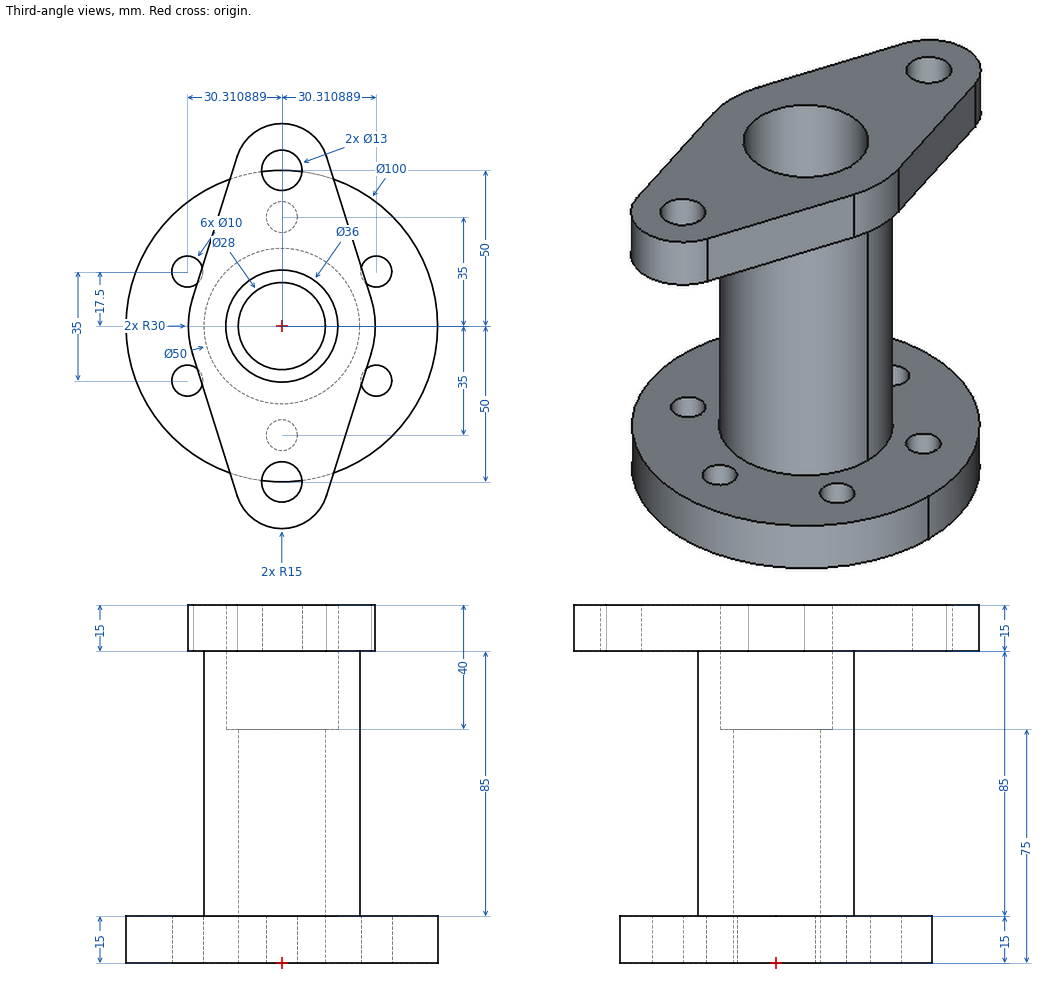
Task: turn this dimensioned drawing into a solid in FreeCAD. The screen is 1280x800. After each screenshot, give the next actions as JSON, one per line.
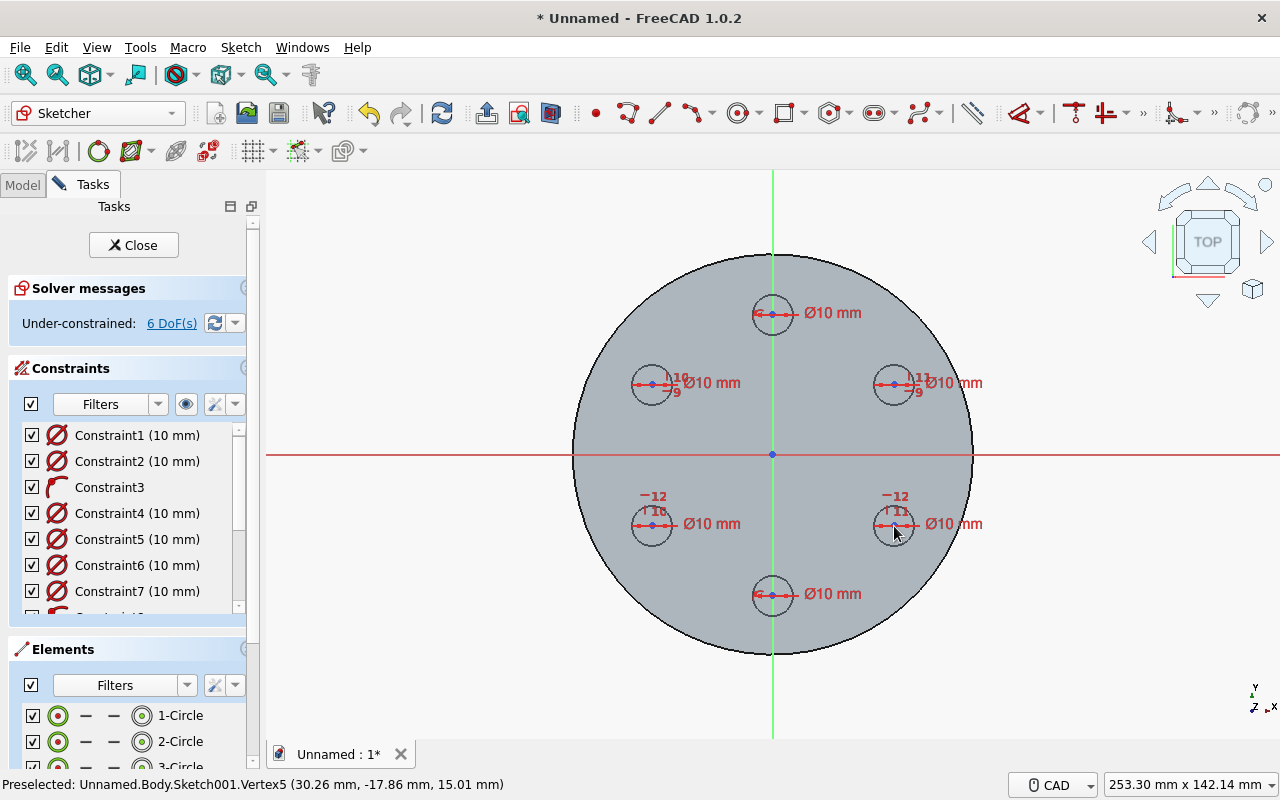
{"action": "left_click", "coordinate": [773, 315]}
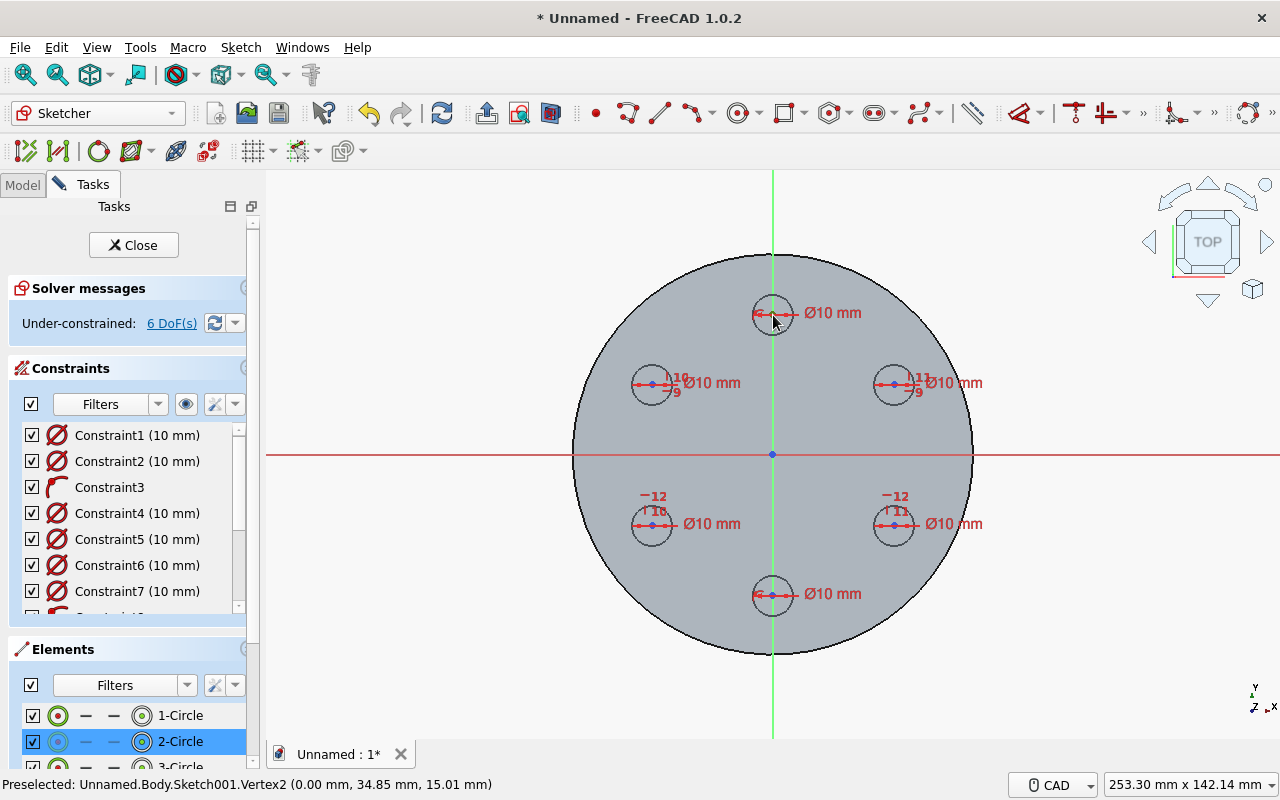
{"action": "key", "text": "i"}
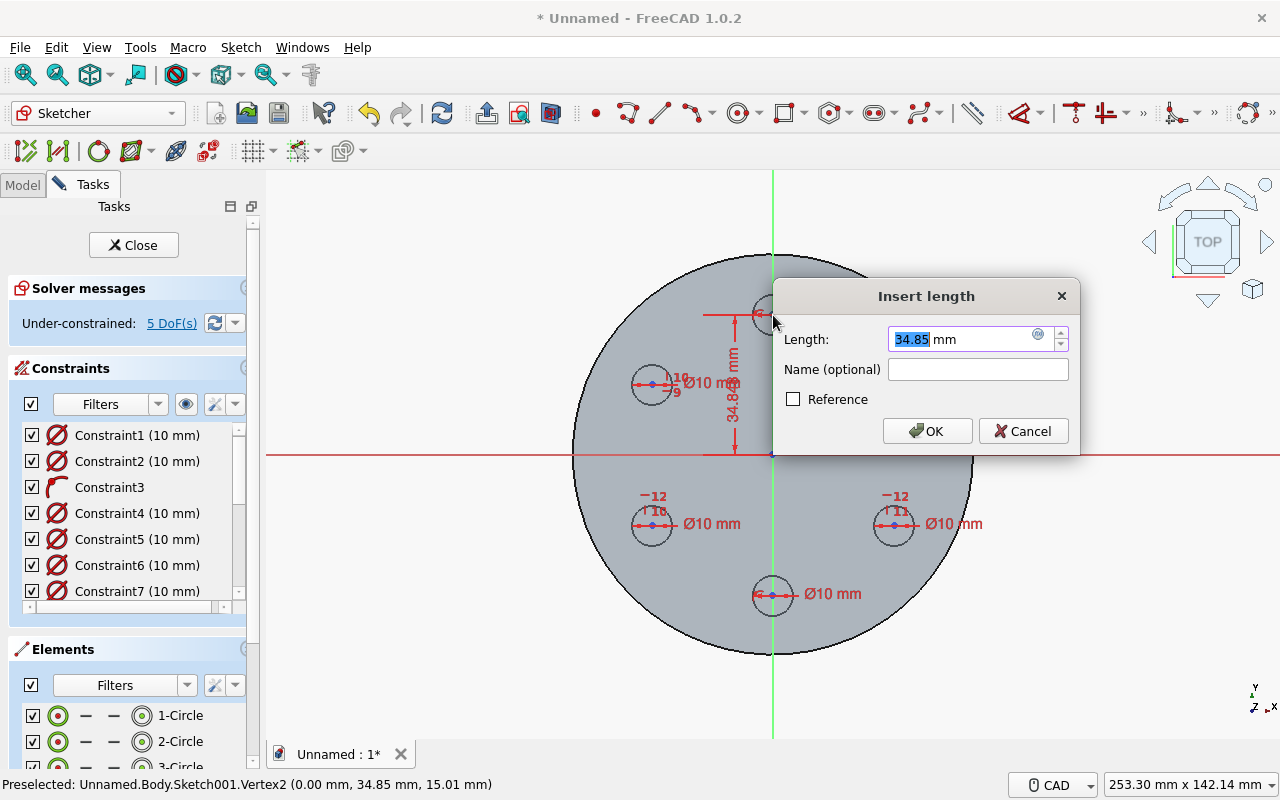
{"action": "type", "text": "35"}
{"action": "key", "text": "Return"}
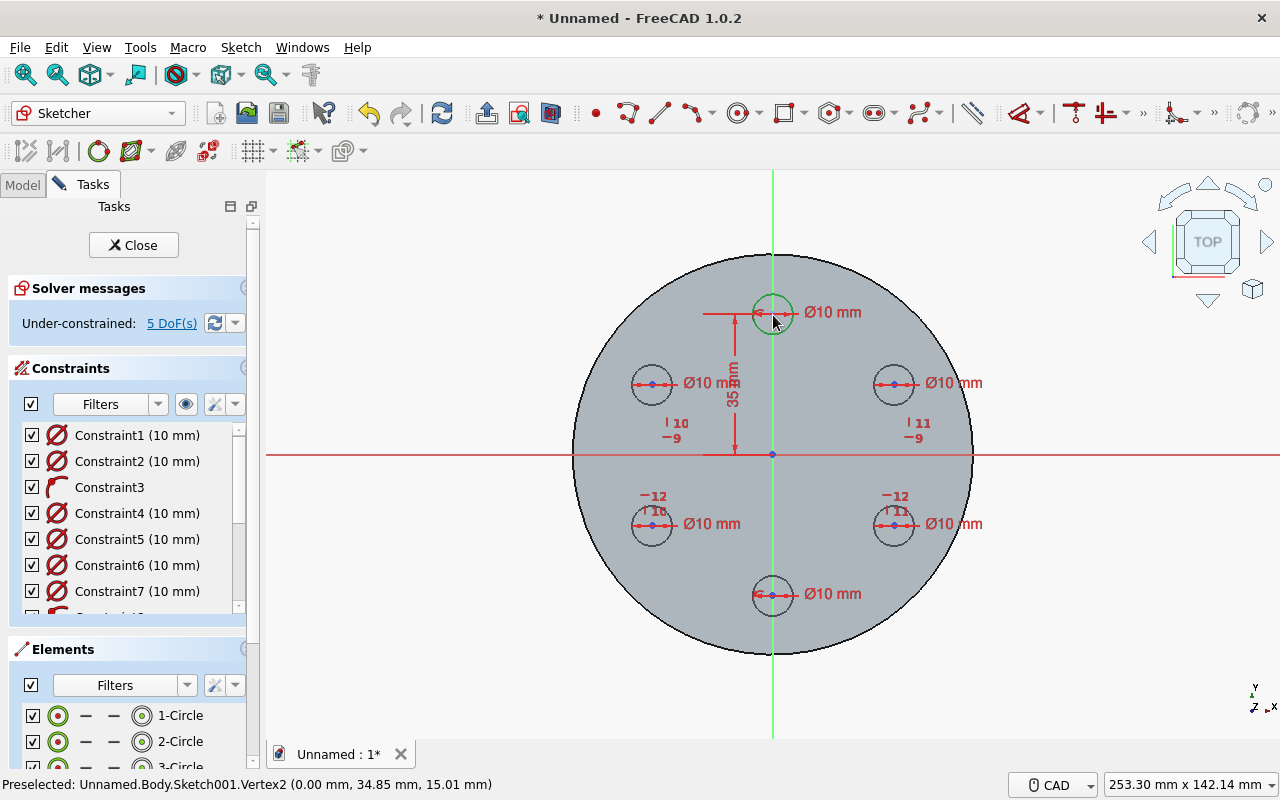
{"action": "left_click", "coordinate": [773, 596]}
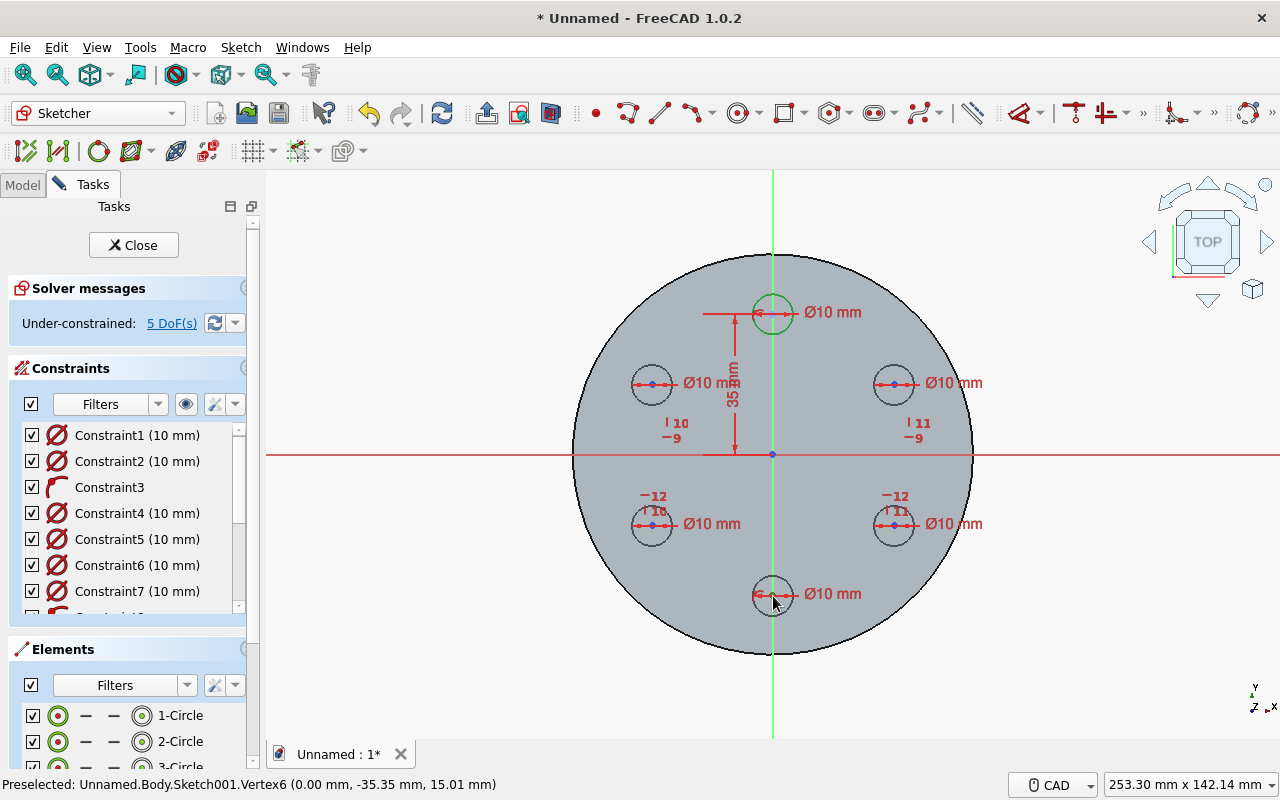
{"action": "key", "text": "i"}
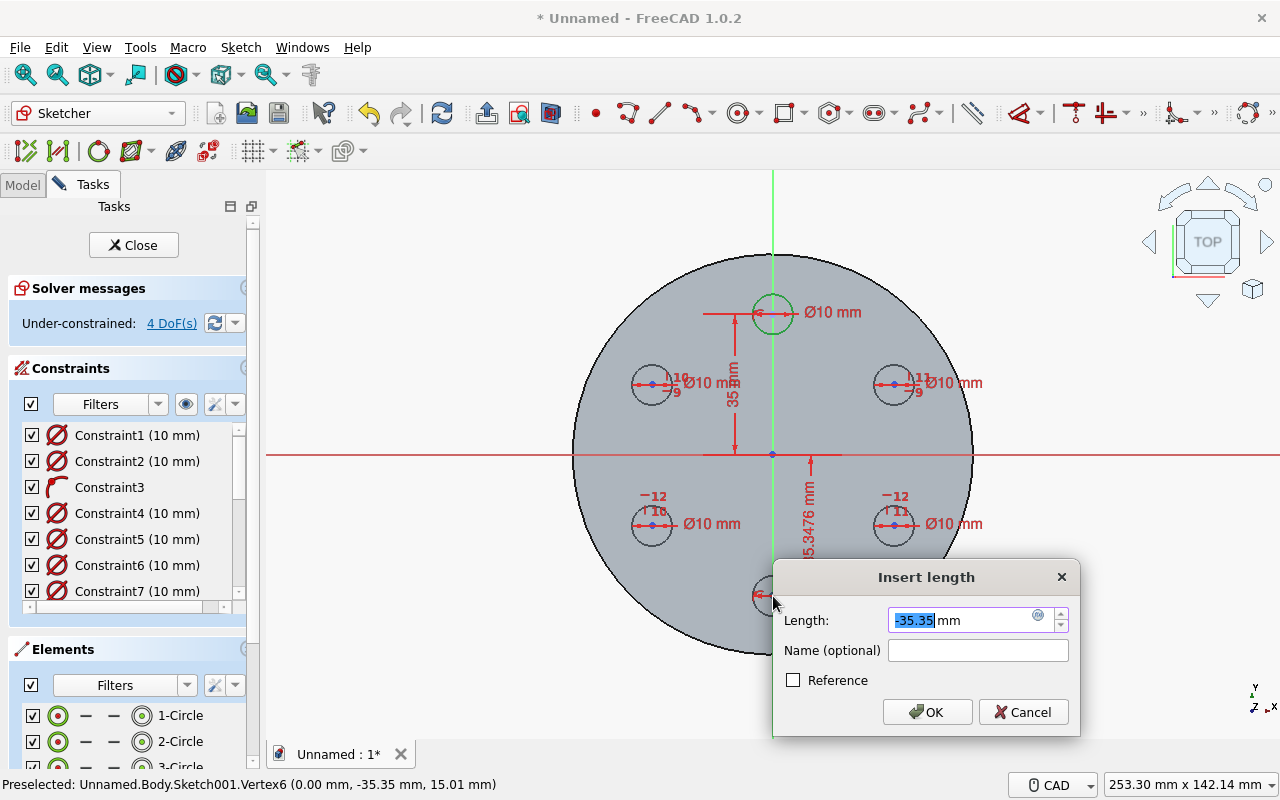
{"action": "type", "text": "-35"}
{"action": "key", "text": "Return"}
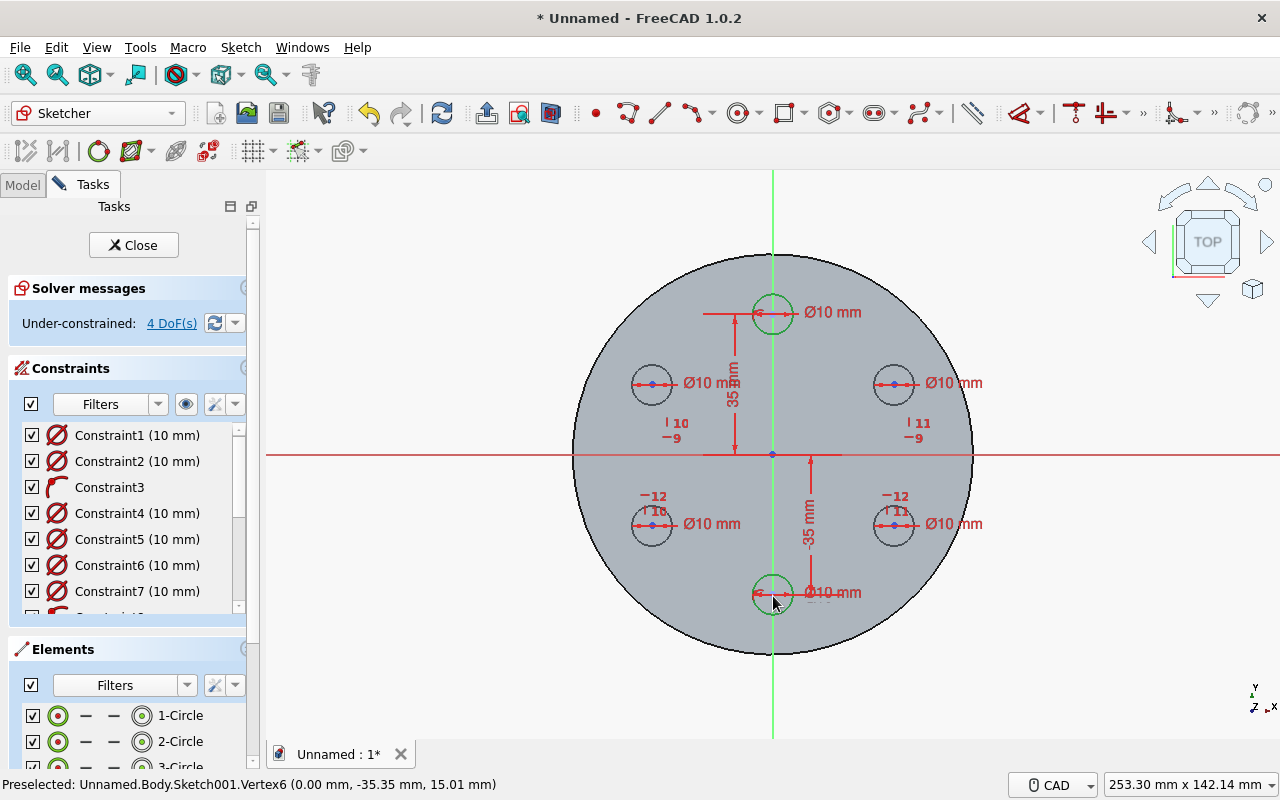
{"action": "left_click", "coordinate": [652, 385]}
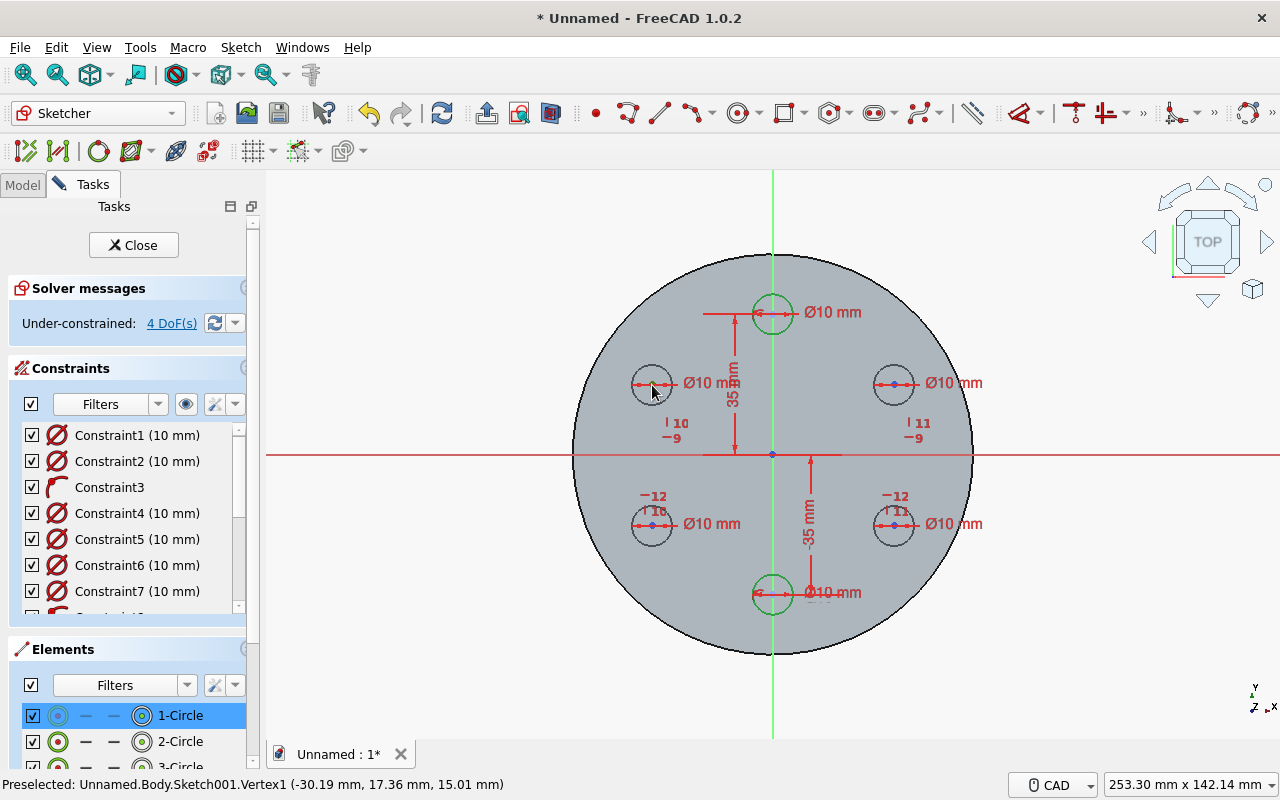
{"action": "left_click", "coordinate": [652, 526]}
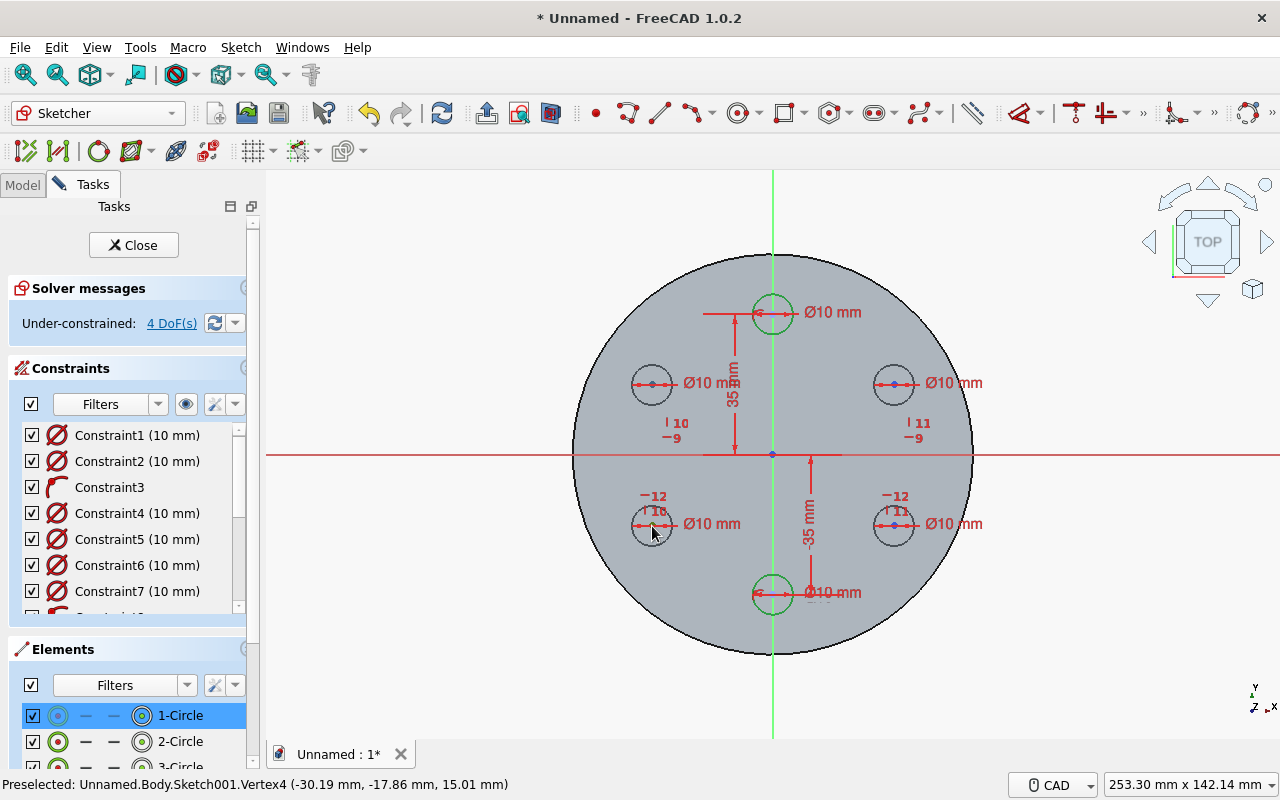
{"action": "key", "text": "i"}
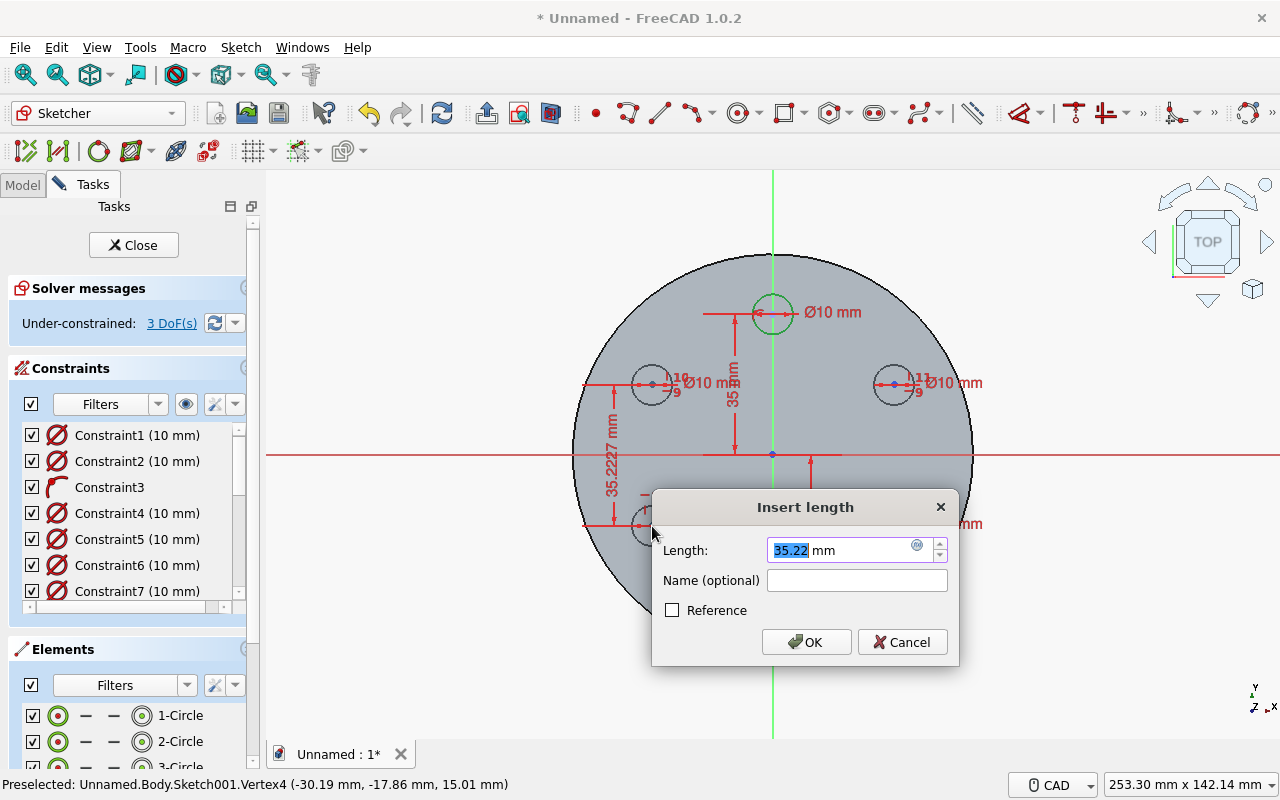
{"action": "type", "text": "35"}
{"action": "key", "text": "Return"}